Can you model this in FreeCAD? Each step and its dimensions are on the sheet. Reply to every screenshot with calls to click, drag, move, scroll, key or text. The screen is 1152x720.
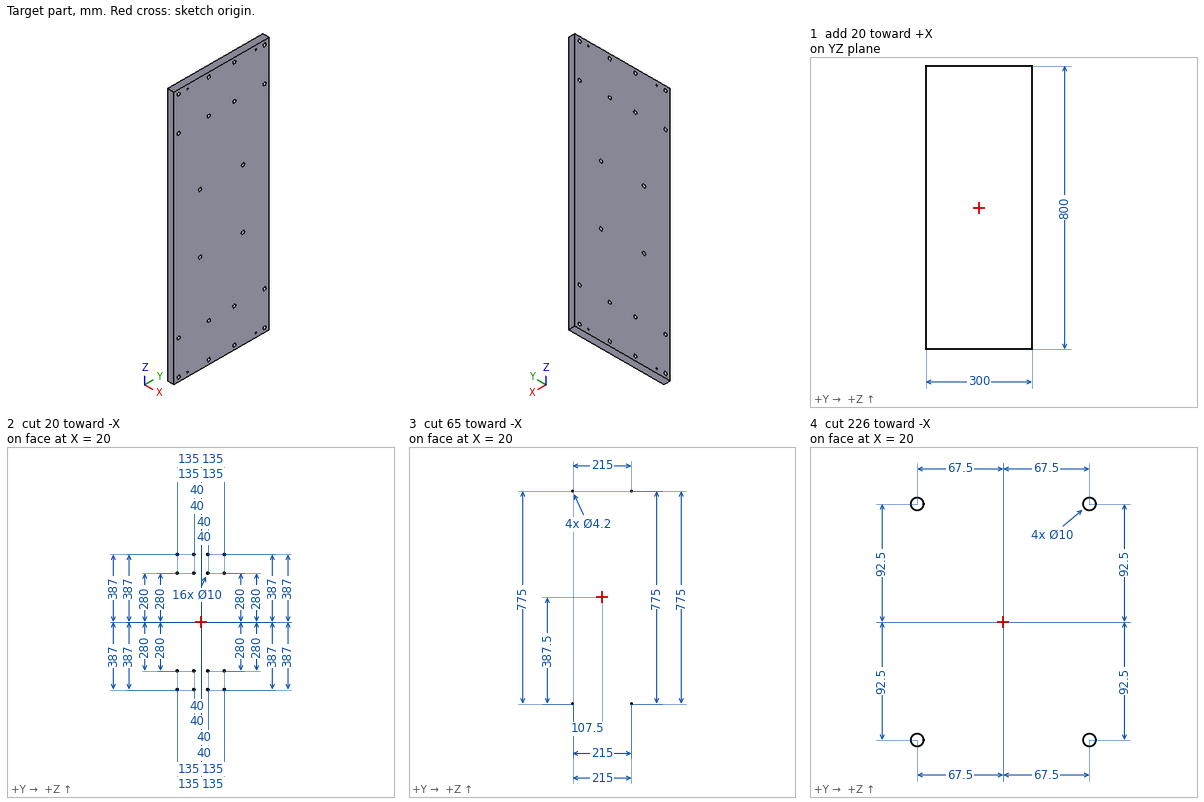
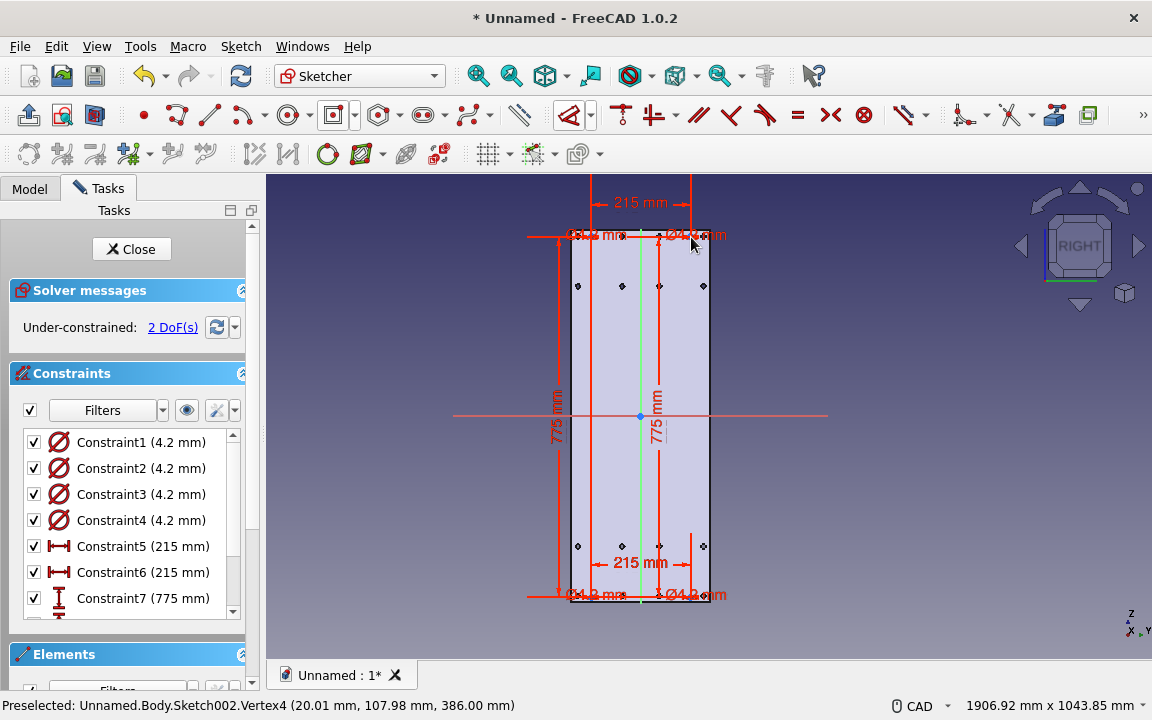
click(591, 597)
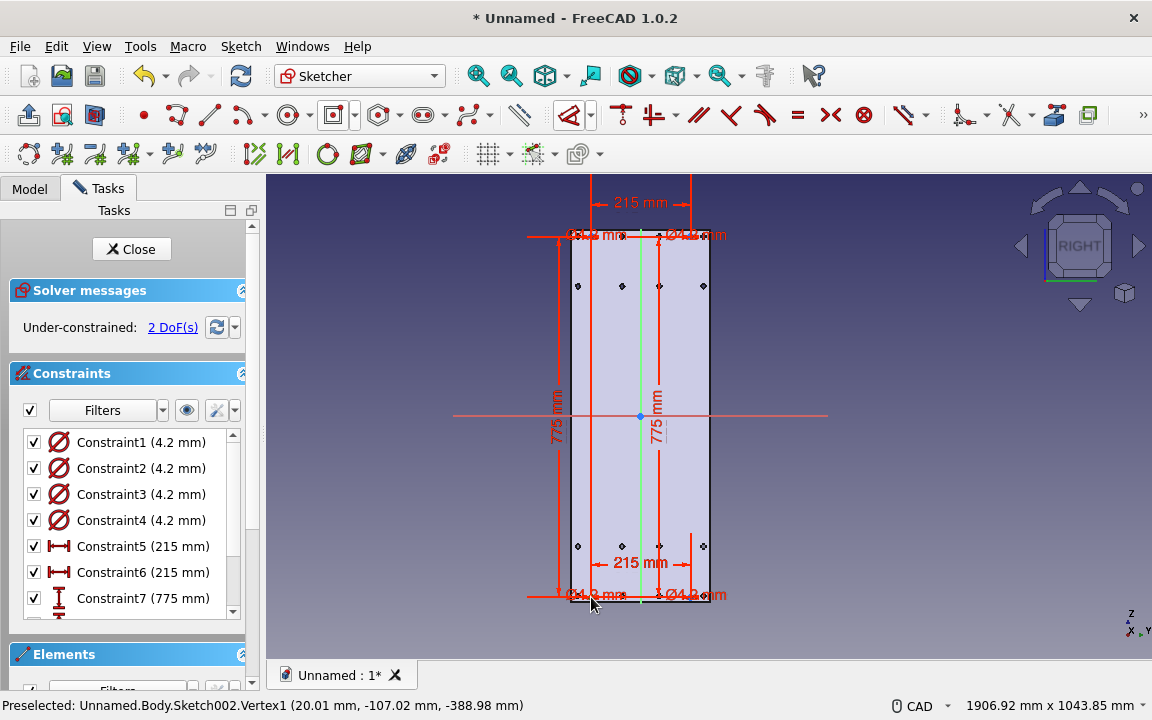
key(l)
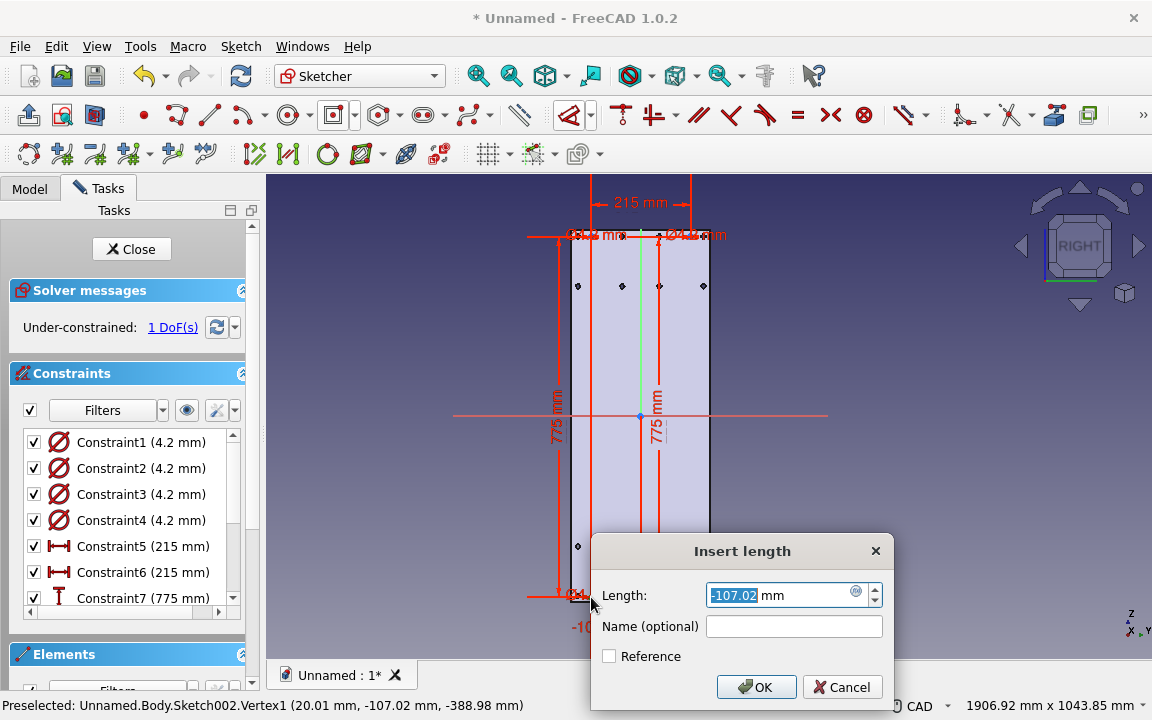
text(-107.5)
key(Return)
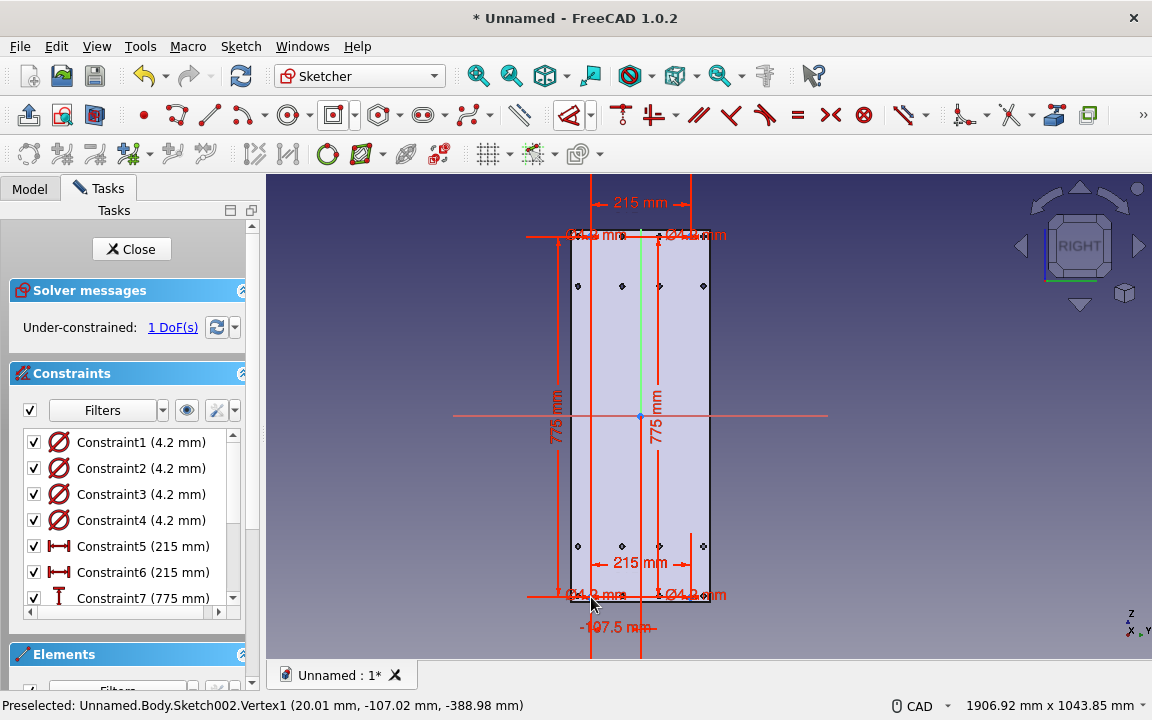
click(591, 597)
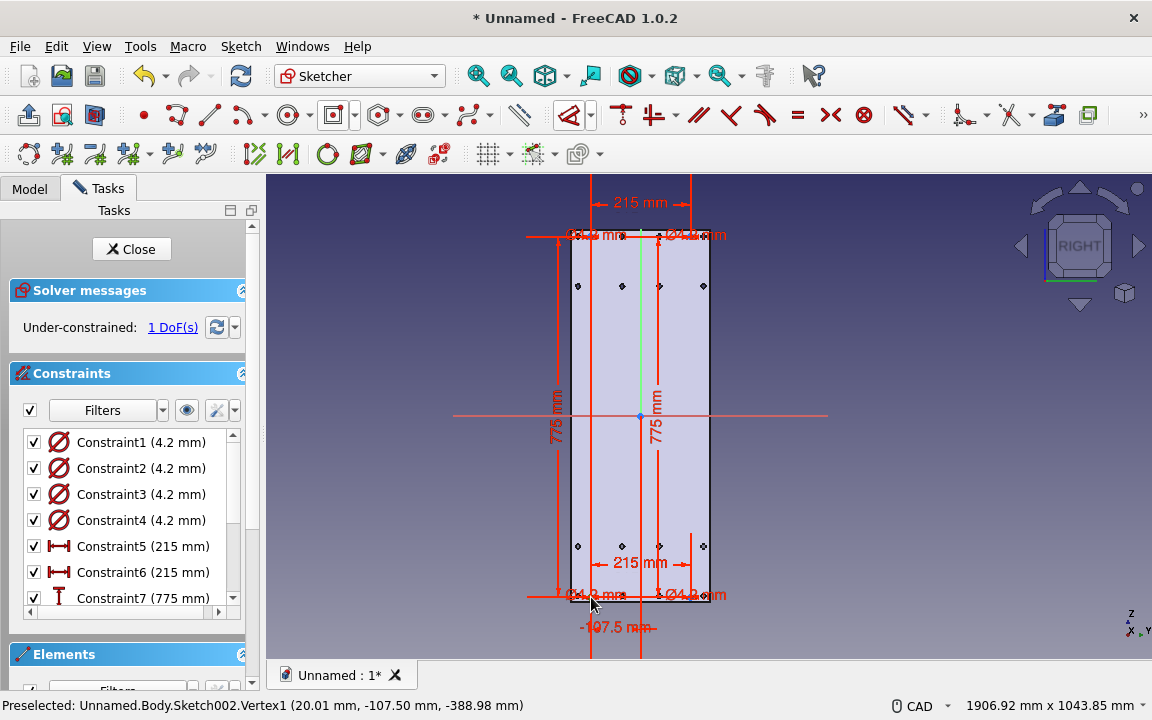
click(590, 116)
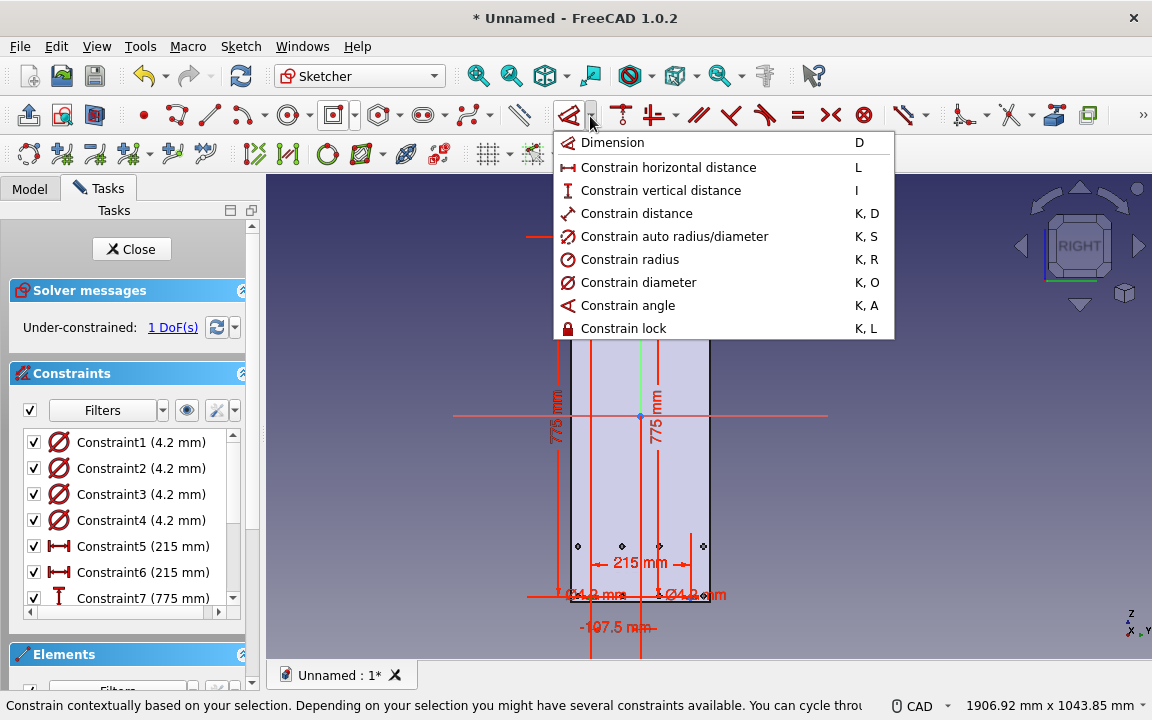
click(724, 190)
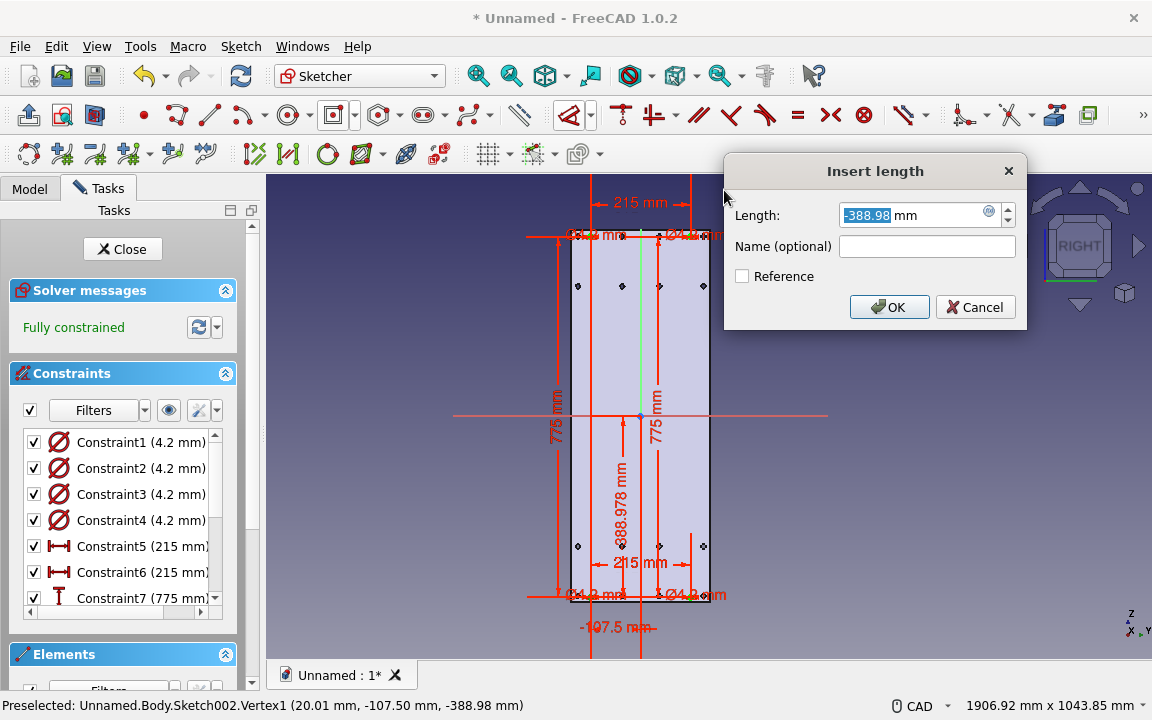
text(-387.5)
key(Return)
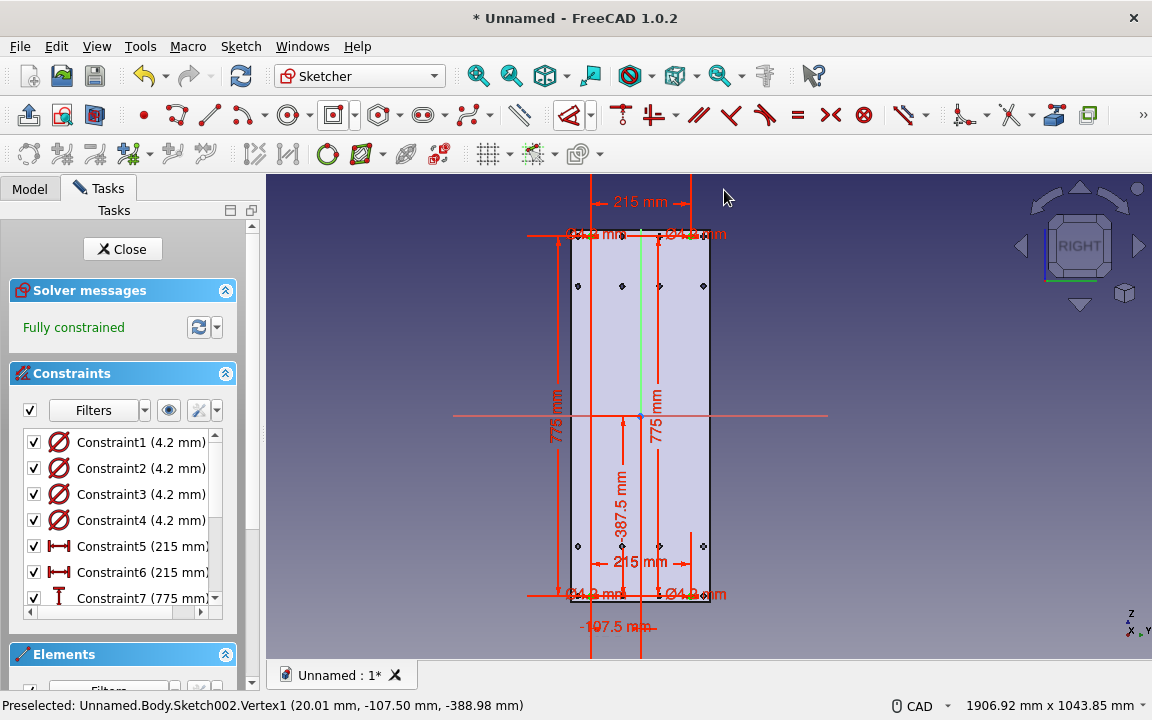
click(123, 249)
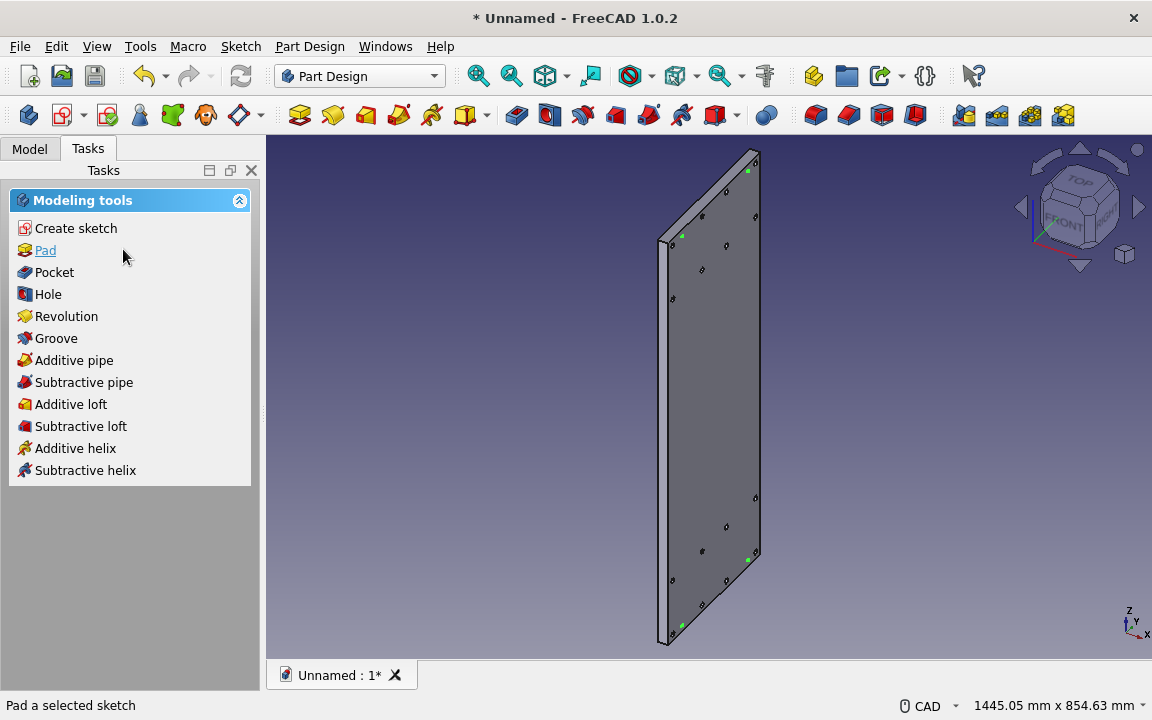
click(517, 116)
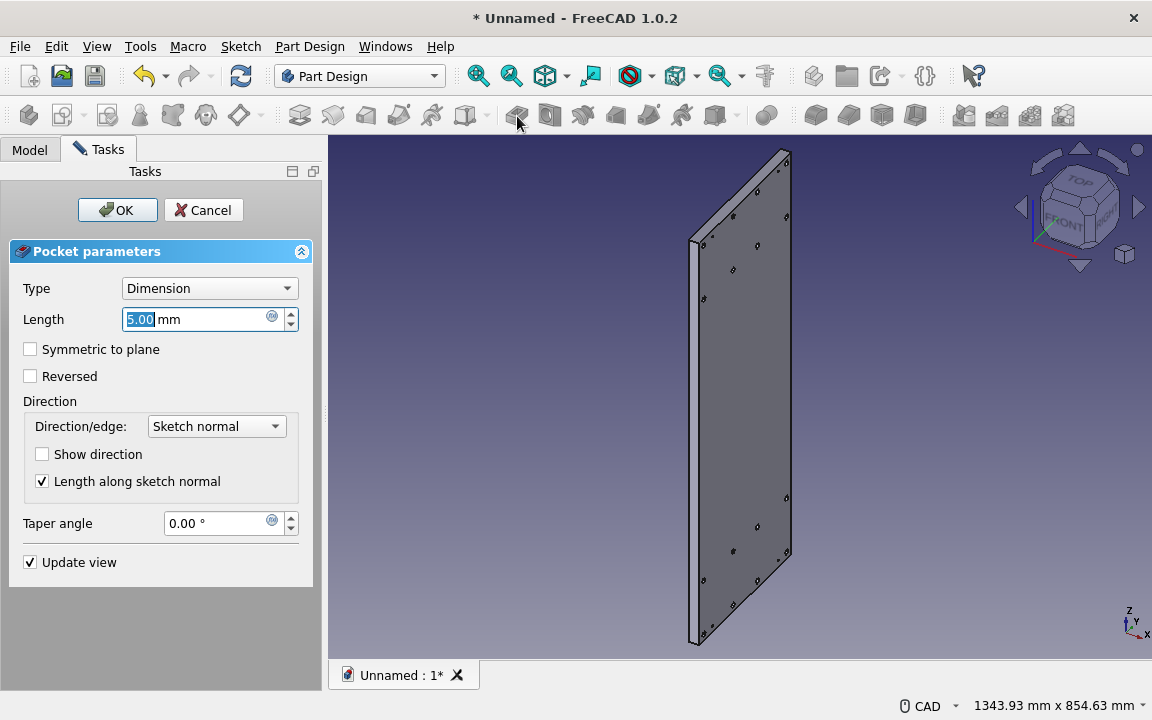
text(65)
key(Tab)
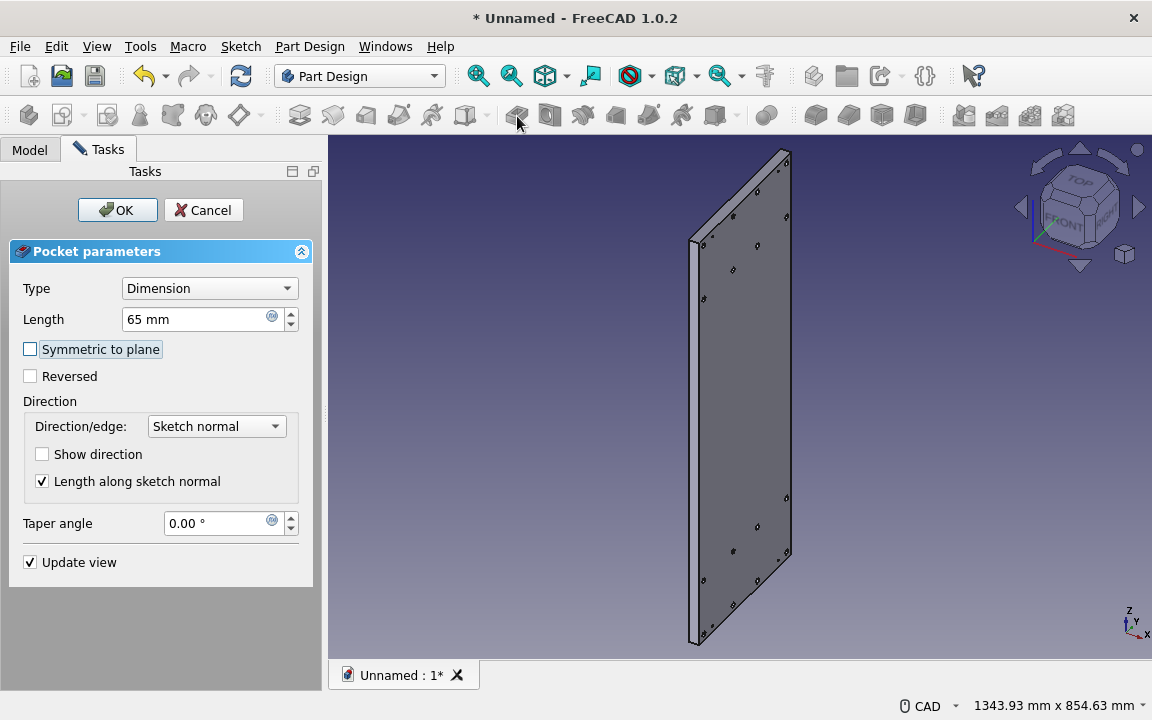
click(118, 210)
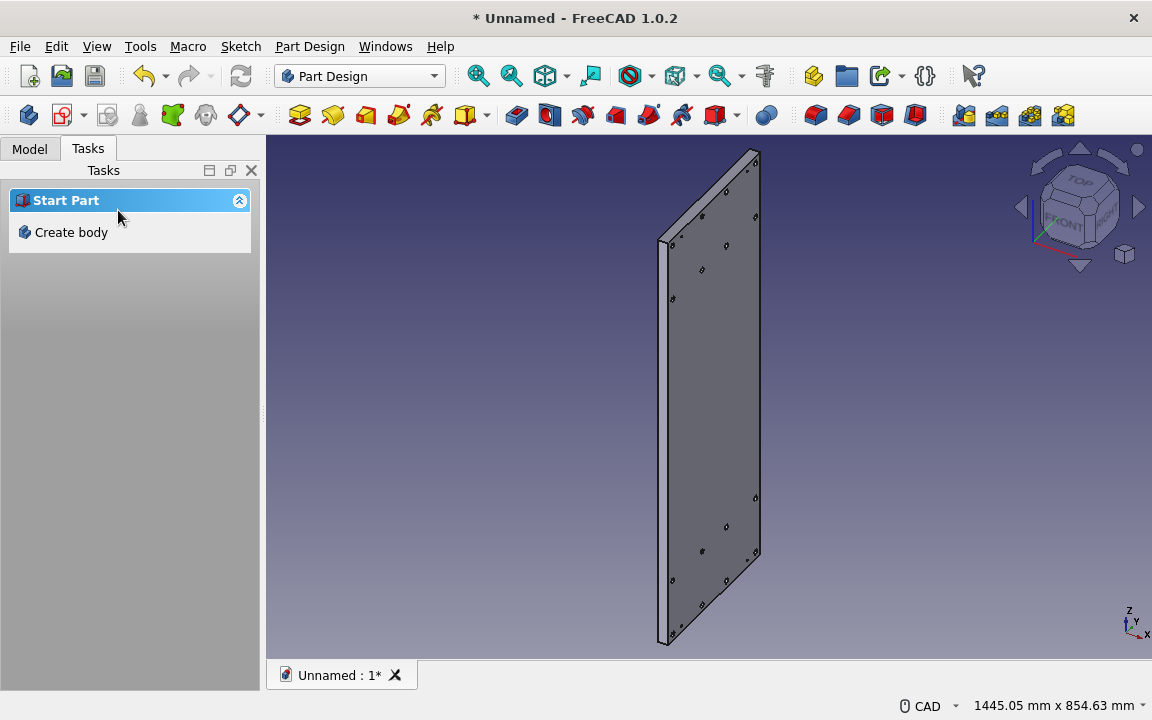
click(714, 398)